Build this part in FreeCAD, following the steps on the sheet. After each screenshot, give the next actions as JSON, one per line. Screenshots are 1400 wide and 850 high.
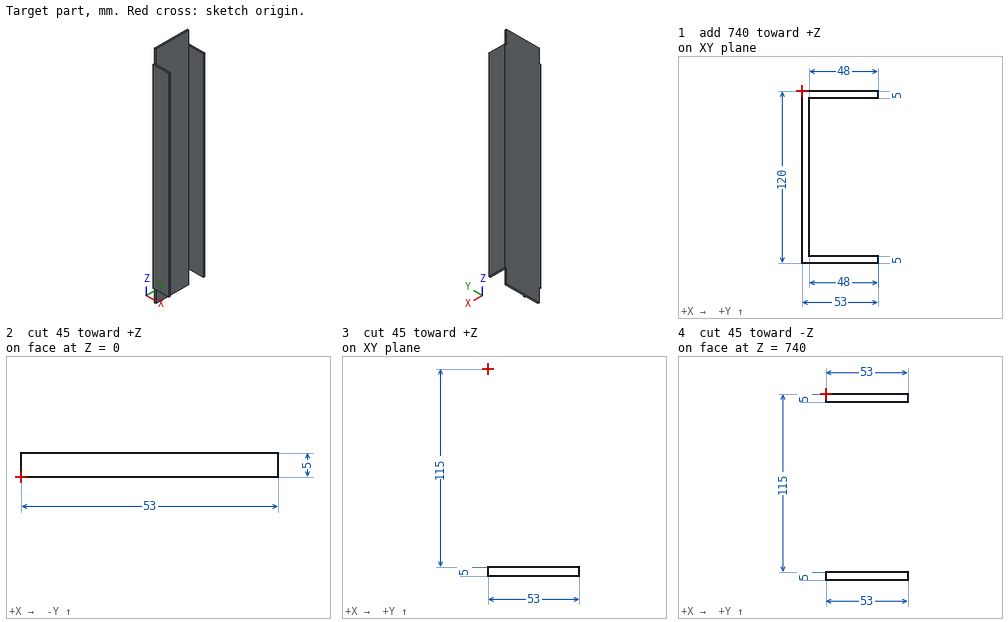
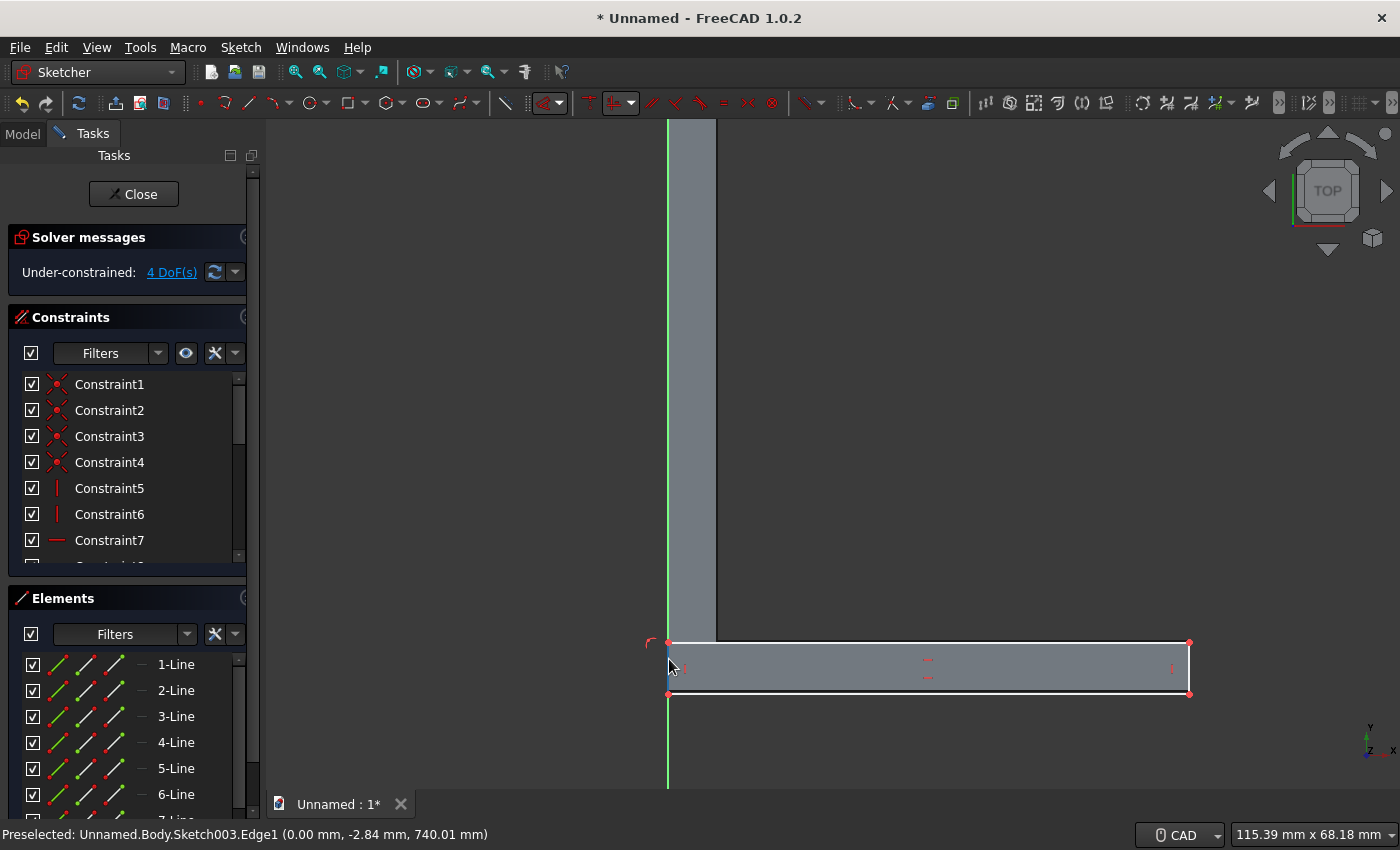
{"action": "left_click", "coordinate": [668, 658]}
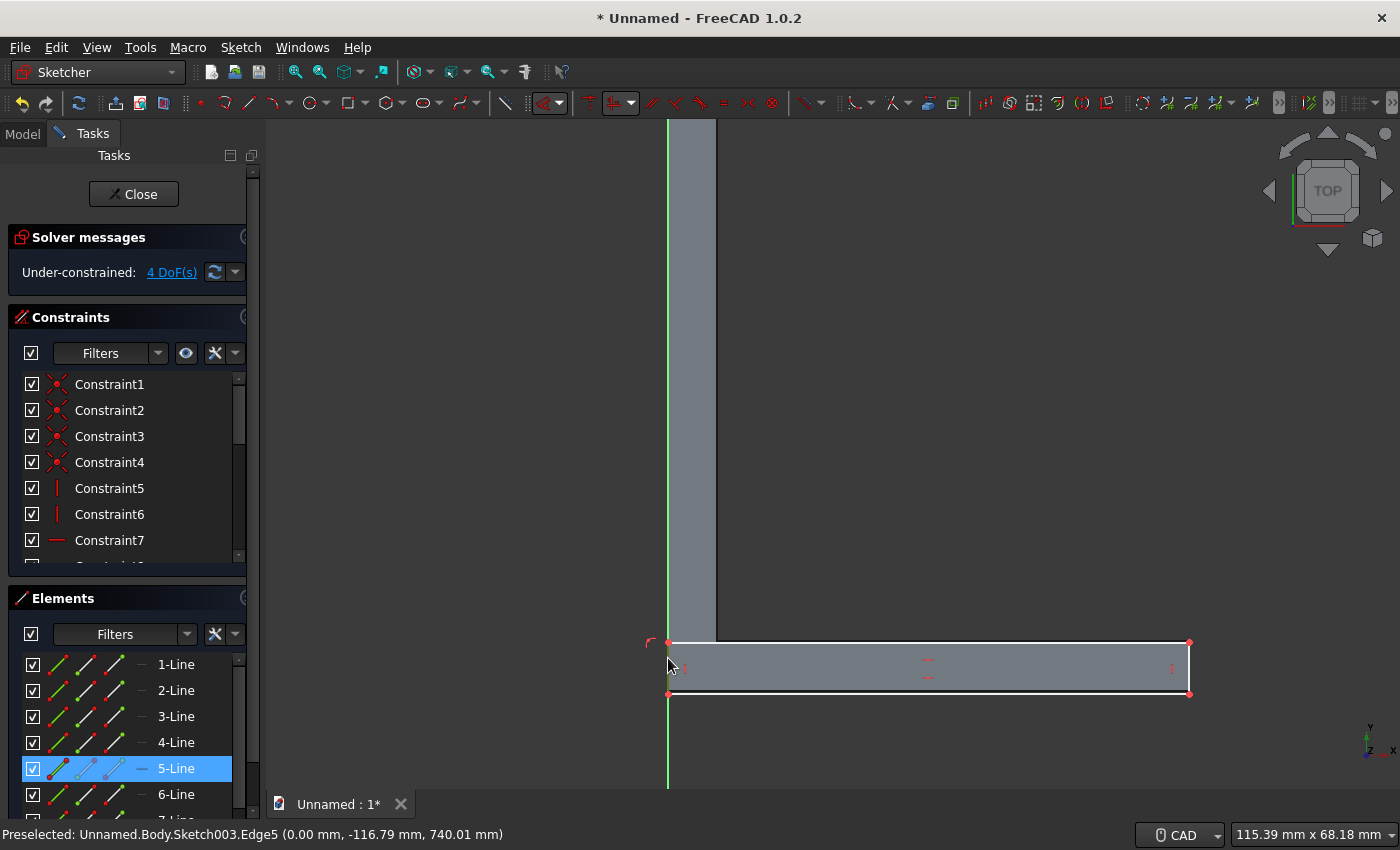
{"action": "key", "text": "i"}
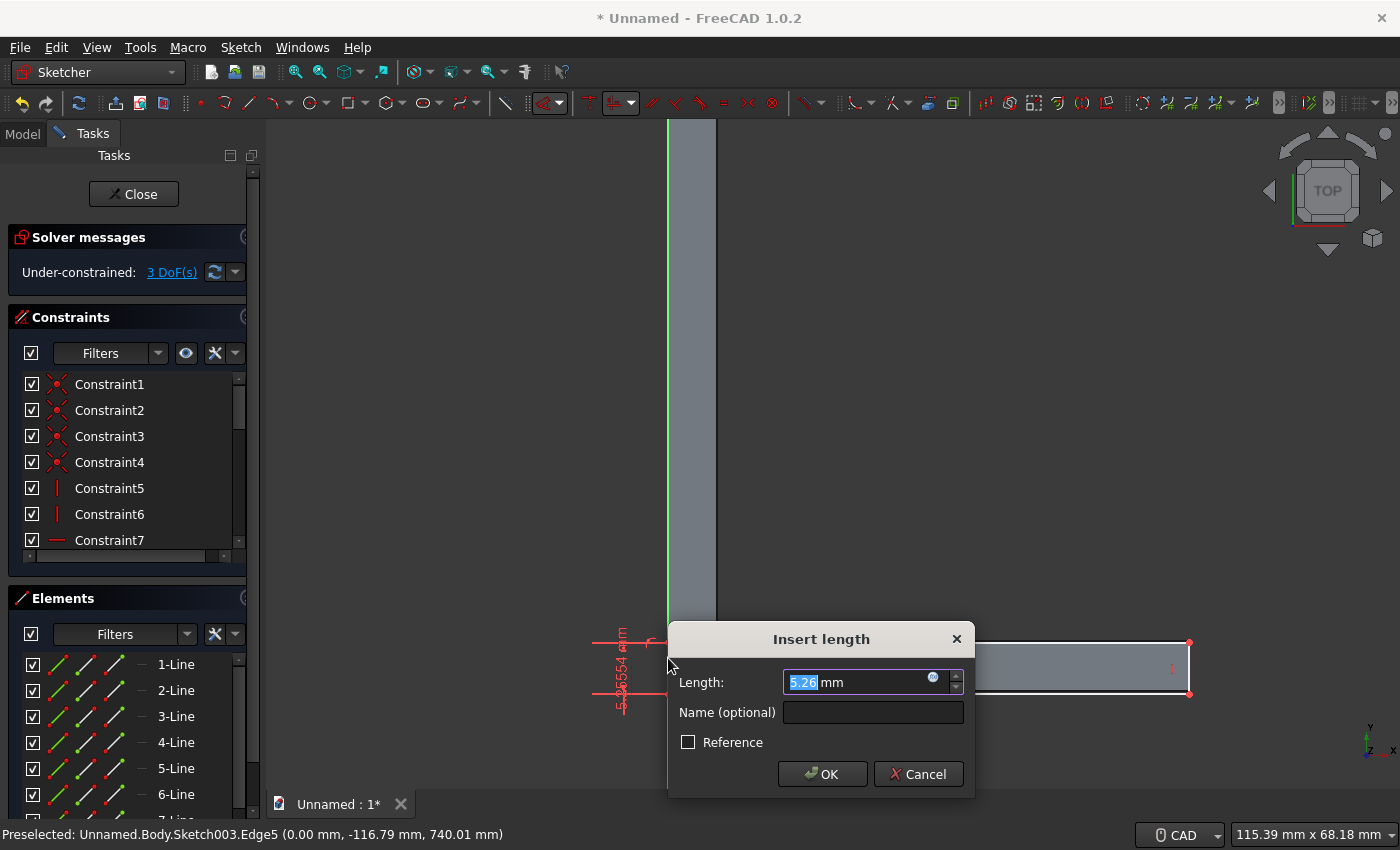
{"action": "type", "text": "5"}
{"action": "key", "text": "Return"}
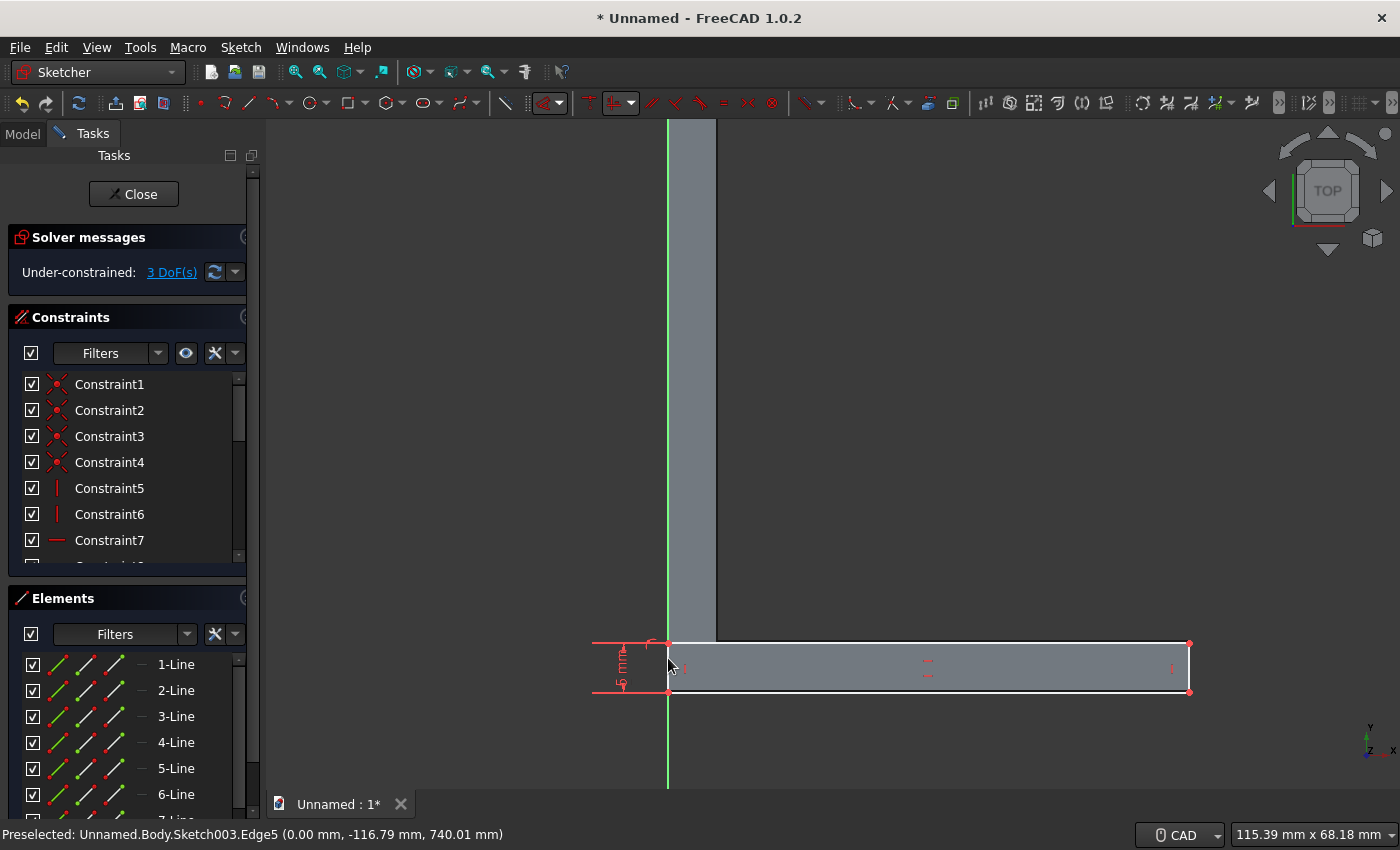
{"action": "scroll", "coordinate": [669, 660], "scroll_direction": "down", "scroll_amount": 5}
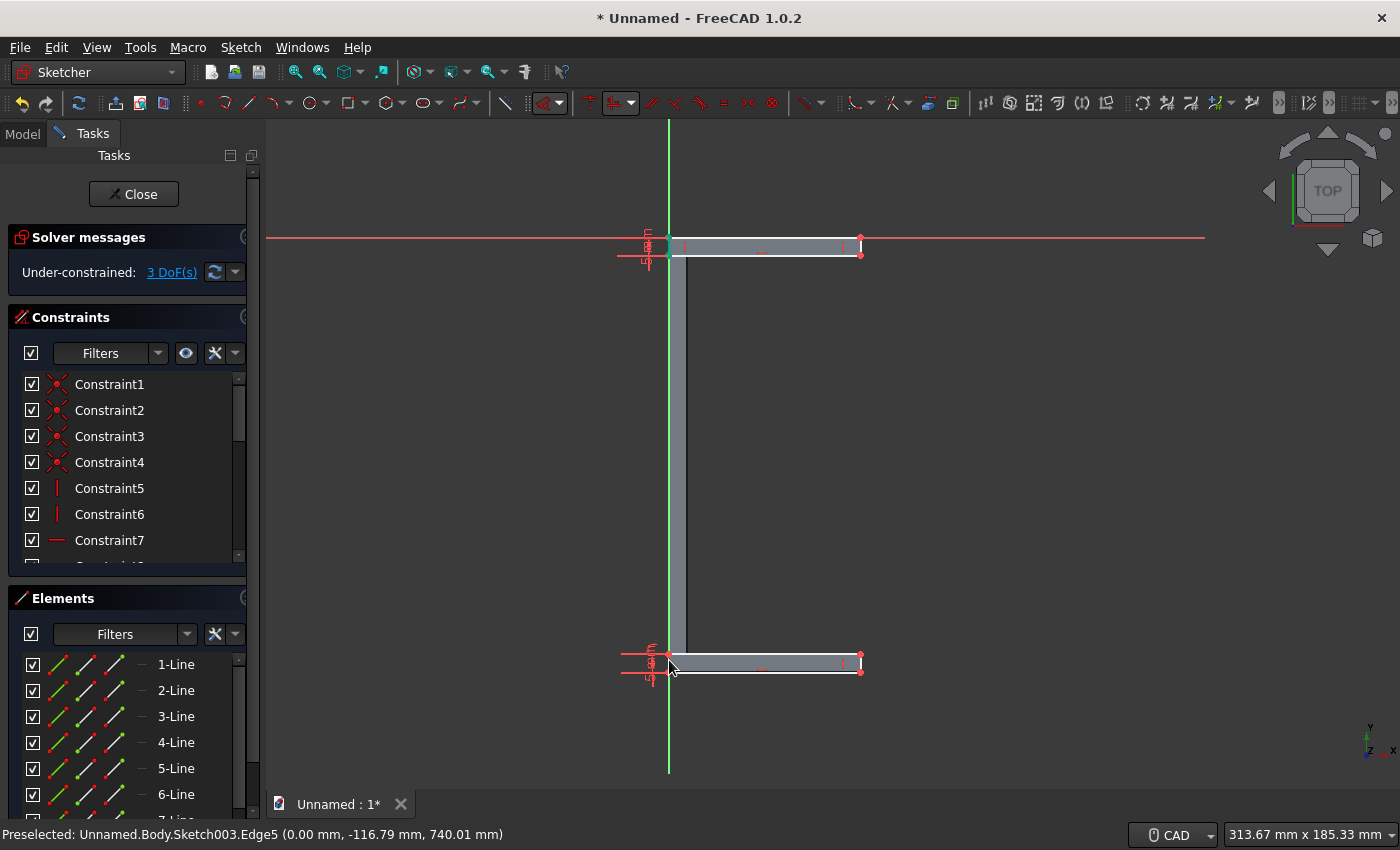
{"action": "left_click", "coordinate": [726, 256]}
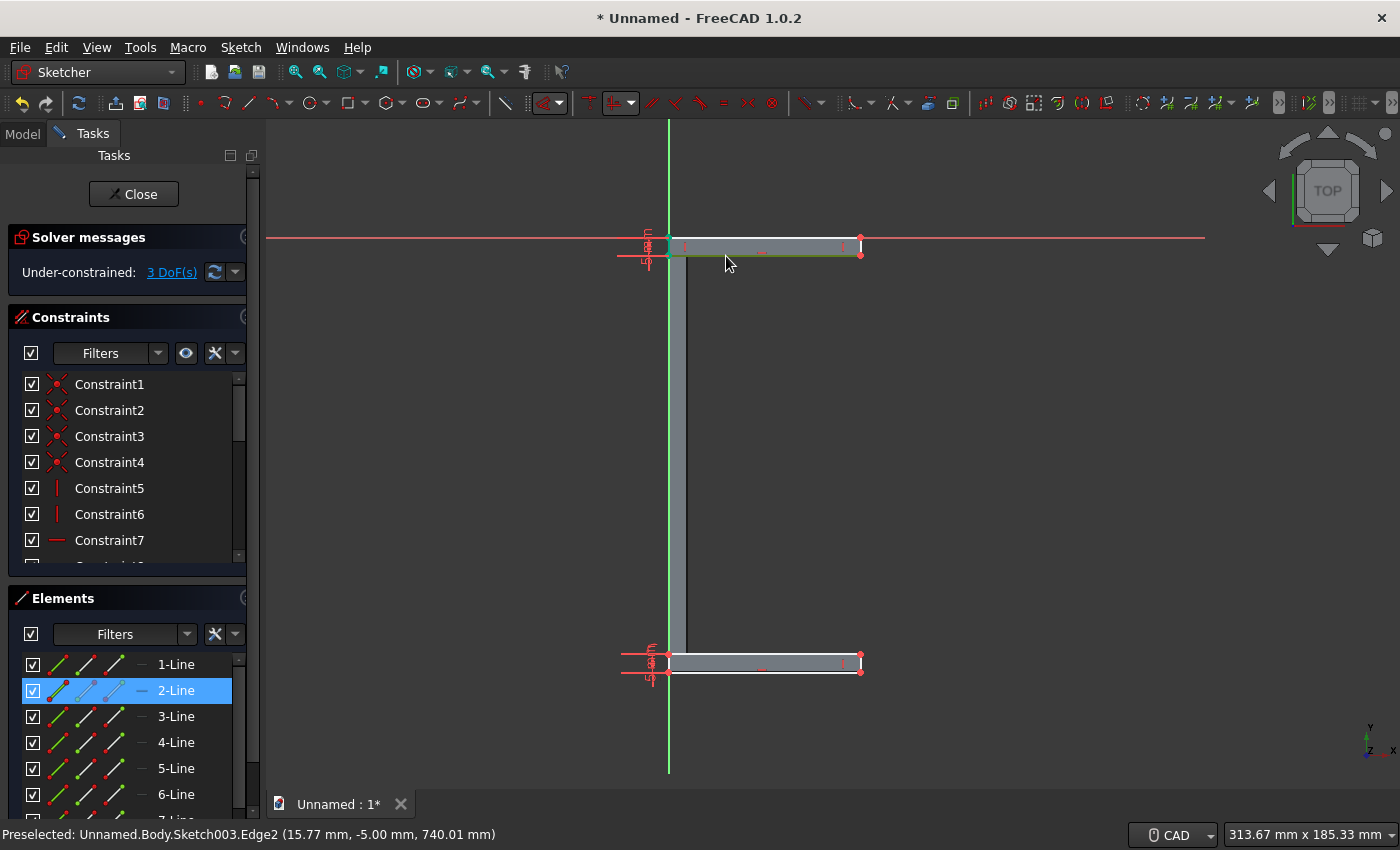
{"action": "key", "text": "l"}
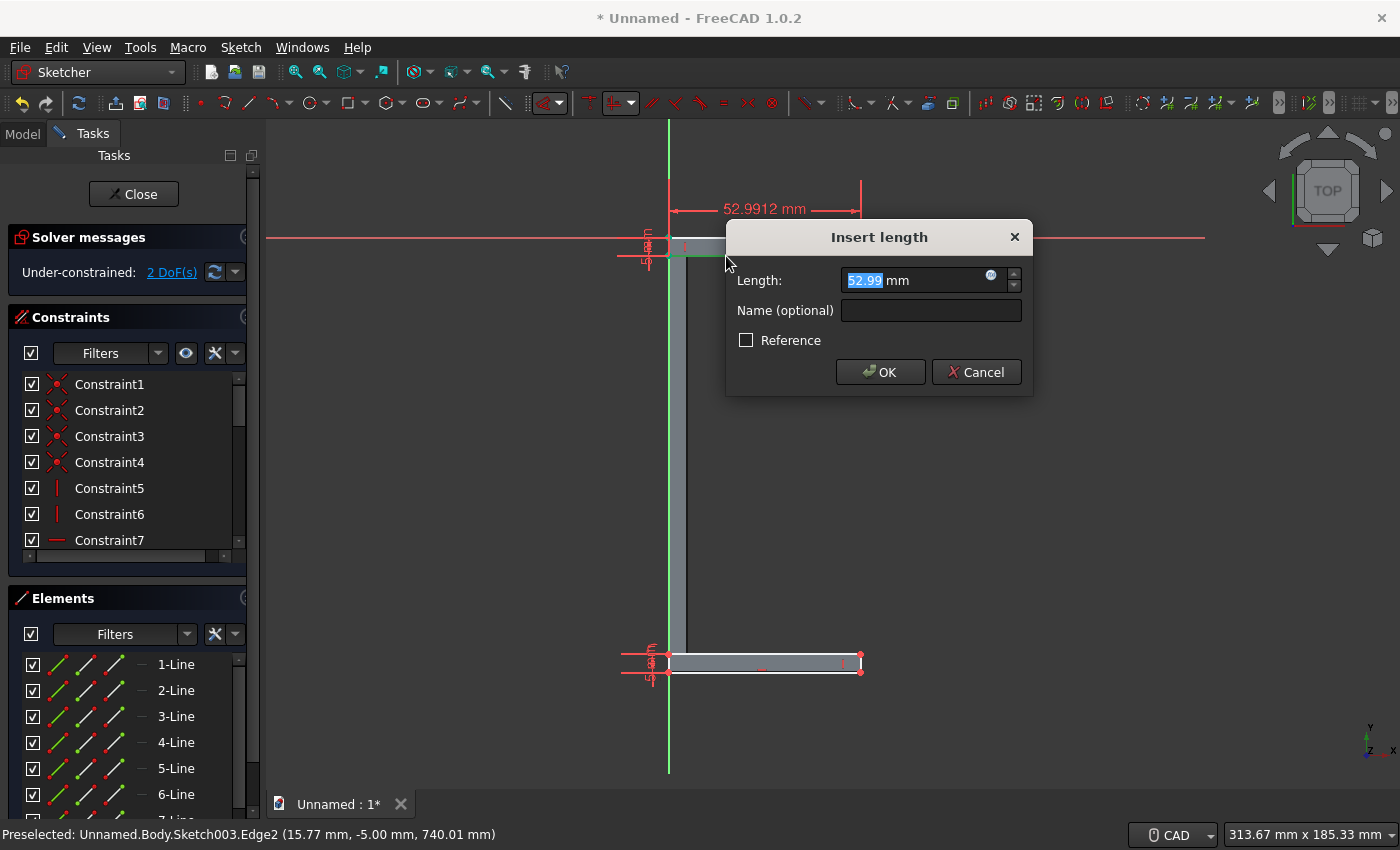
{"action": "type", "text": "53"}
{"action": "key", "text": "Return"}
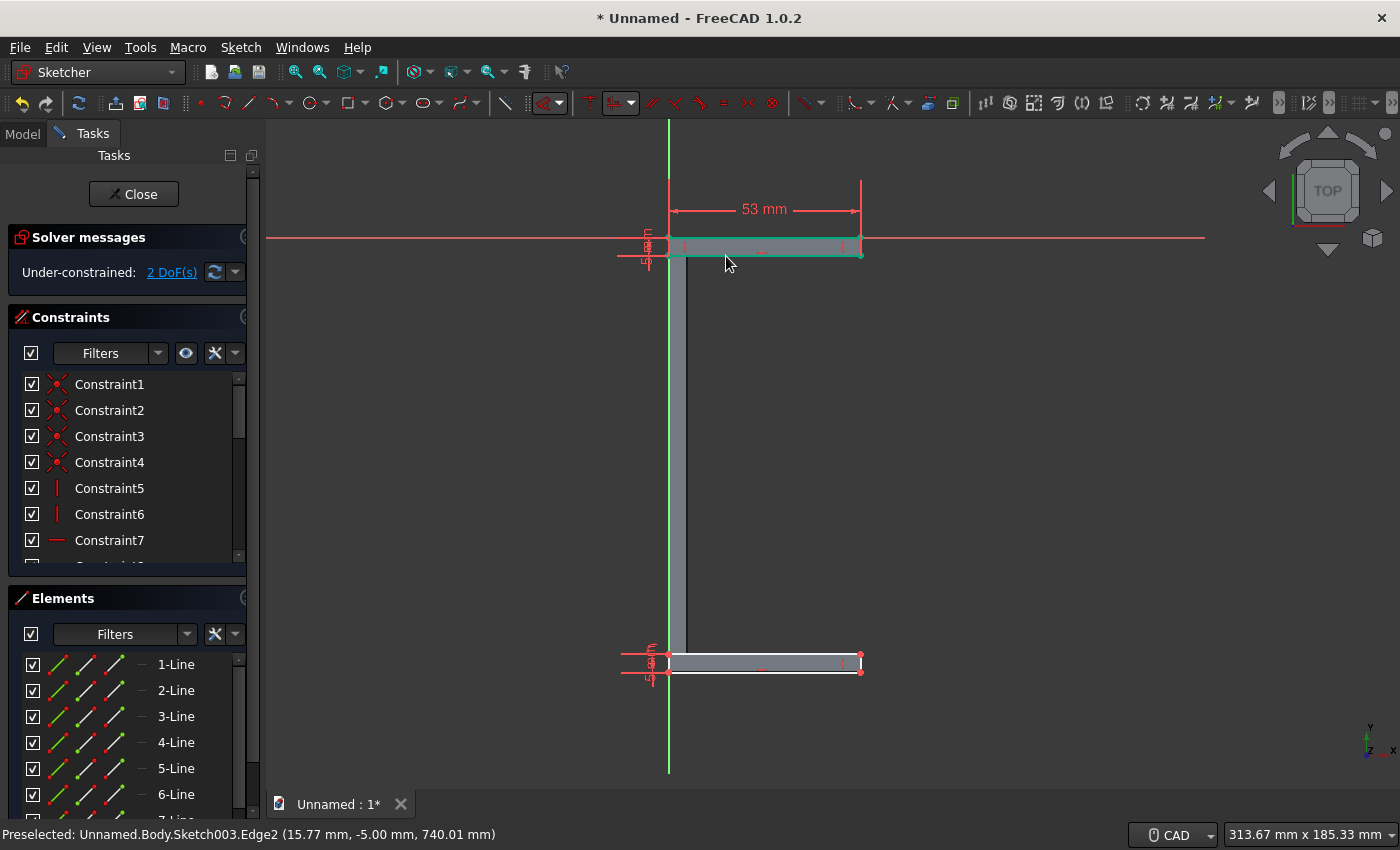
{"action": "left_click", "coordinate": [726, 673]}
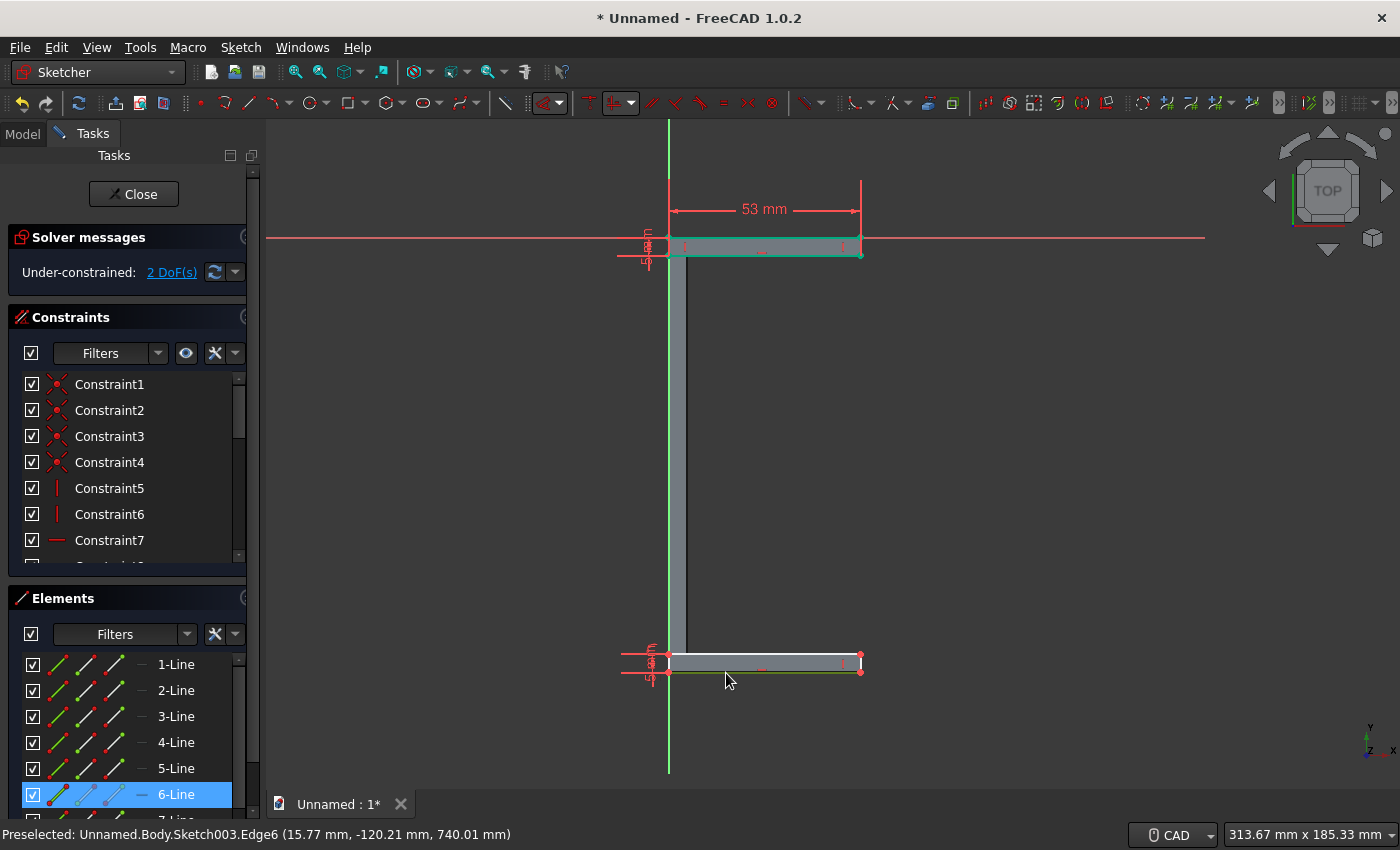
{"action": "left_click", "coordinate": [562, 104]}